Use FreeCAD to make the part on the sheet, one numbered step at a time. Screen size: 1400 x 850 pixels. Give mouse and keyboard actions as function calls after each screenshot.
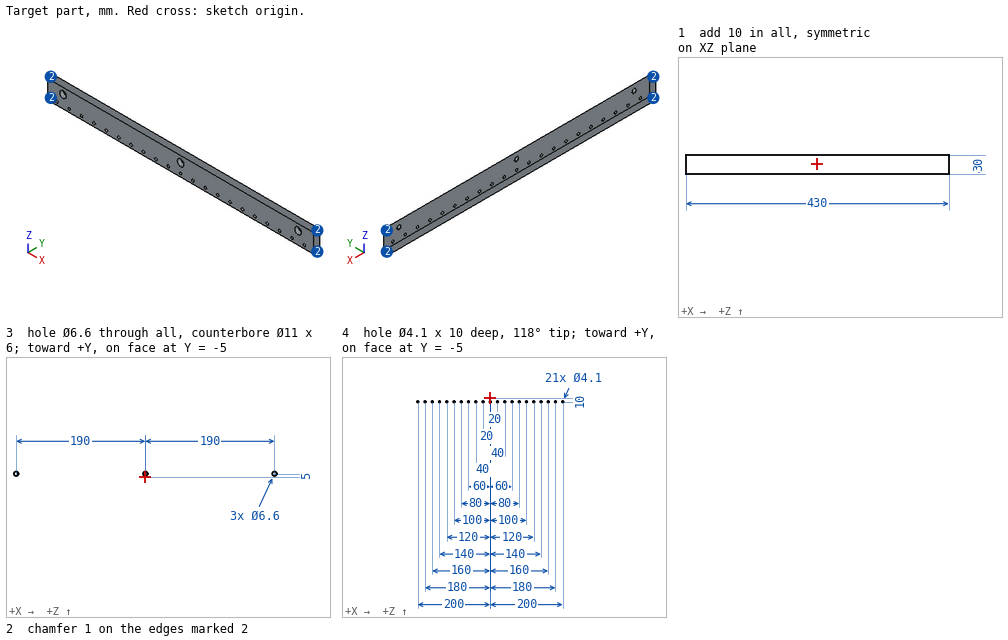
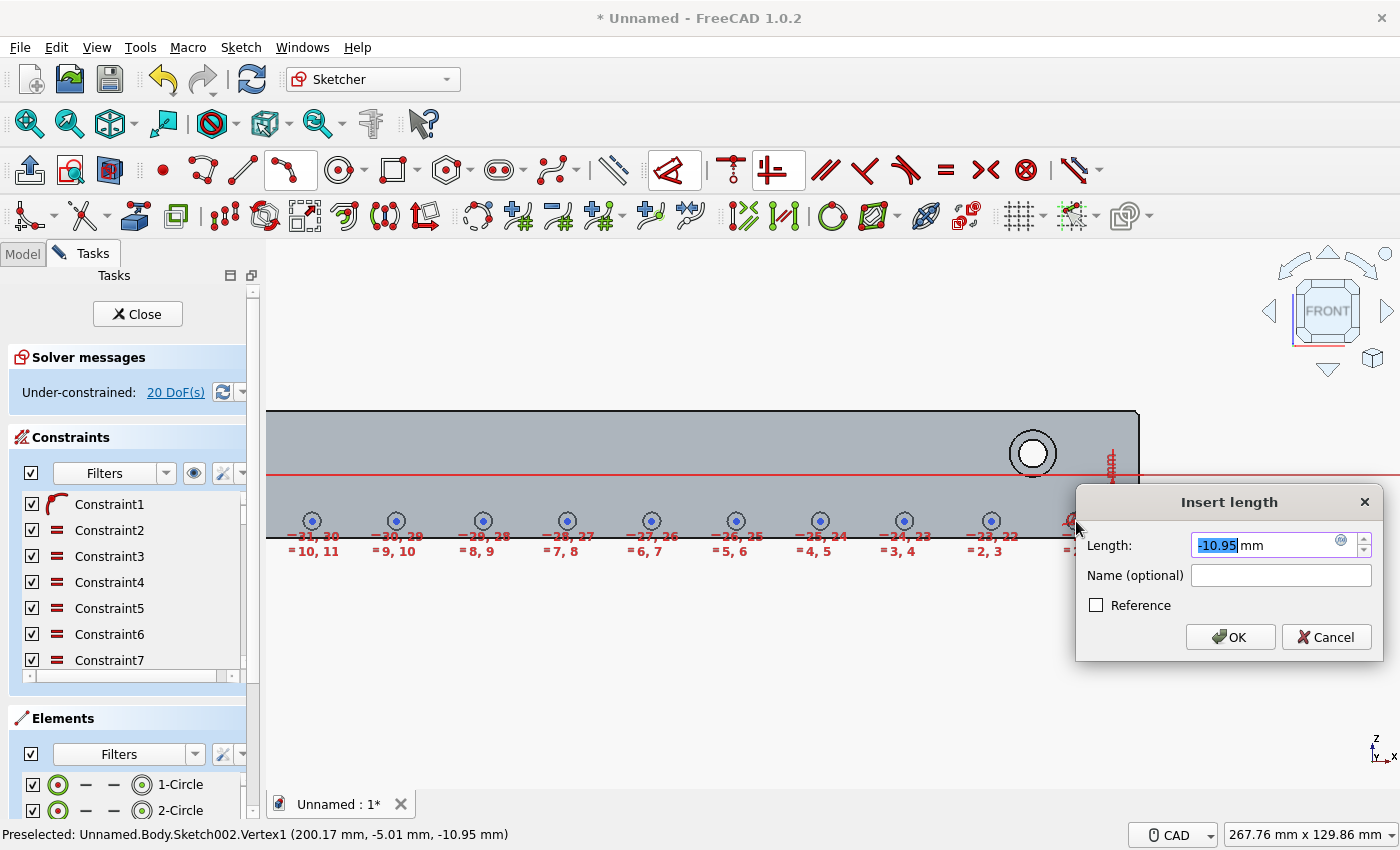
text(-10)
key(Return)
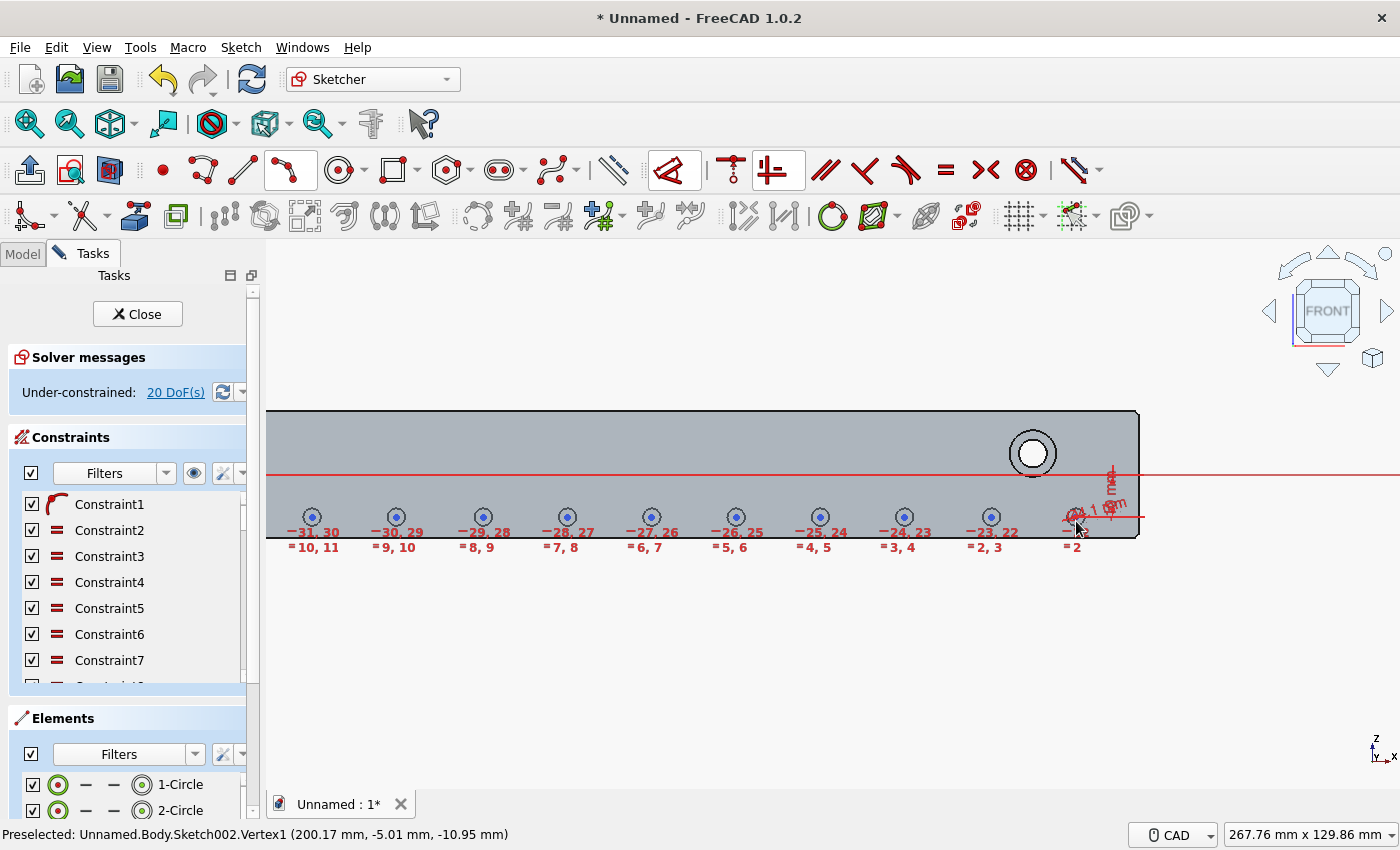
click(568, 517)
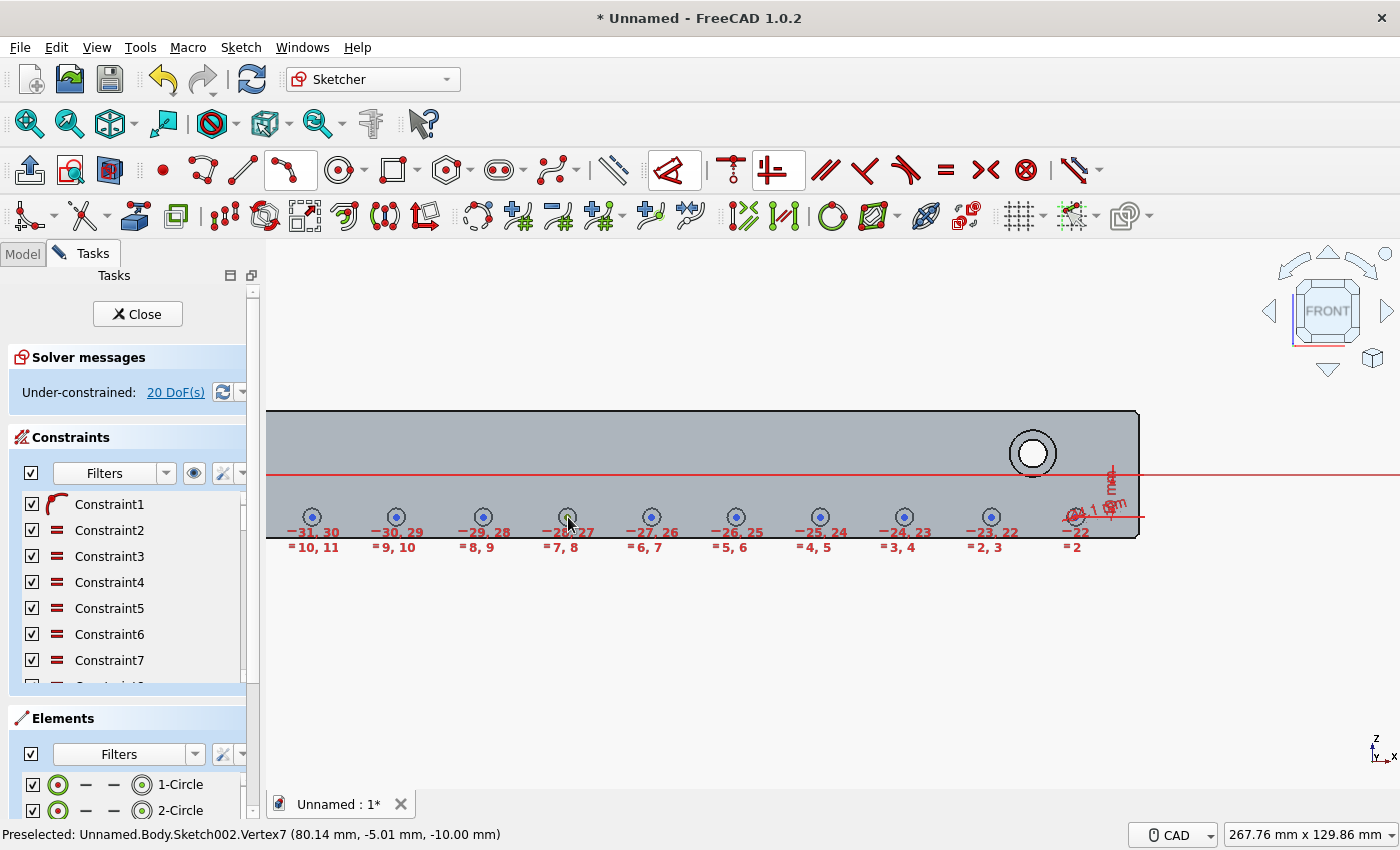
key(l)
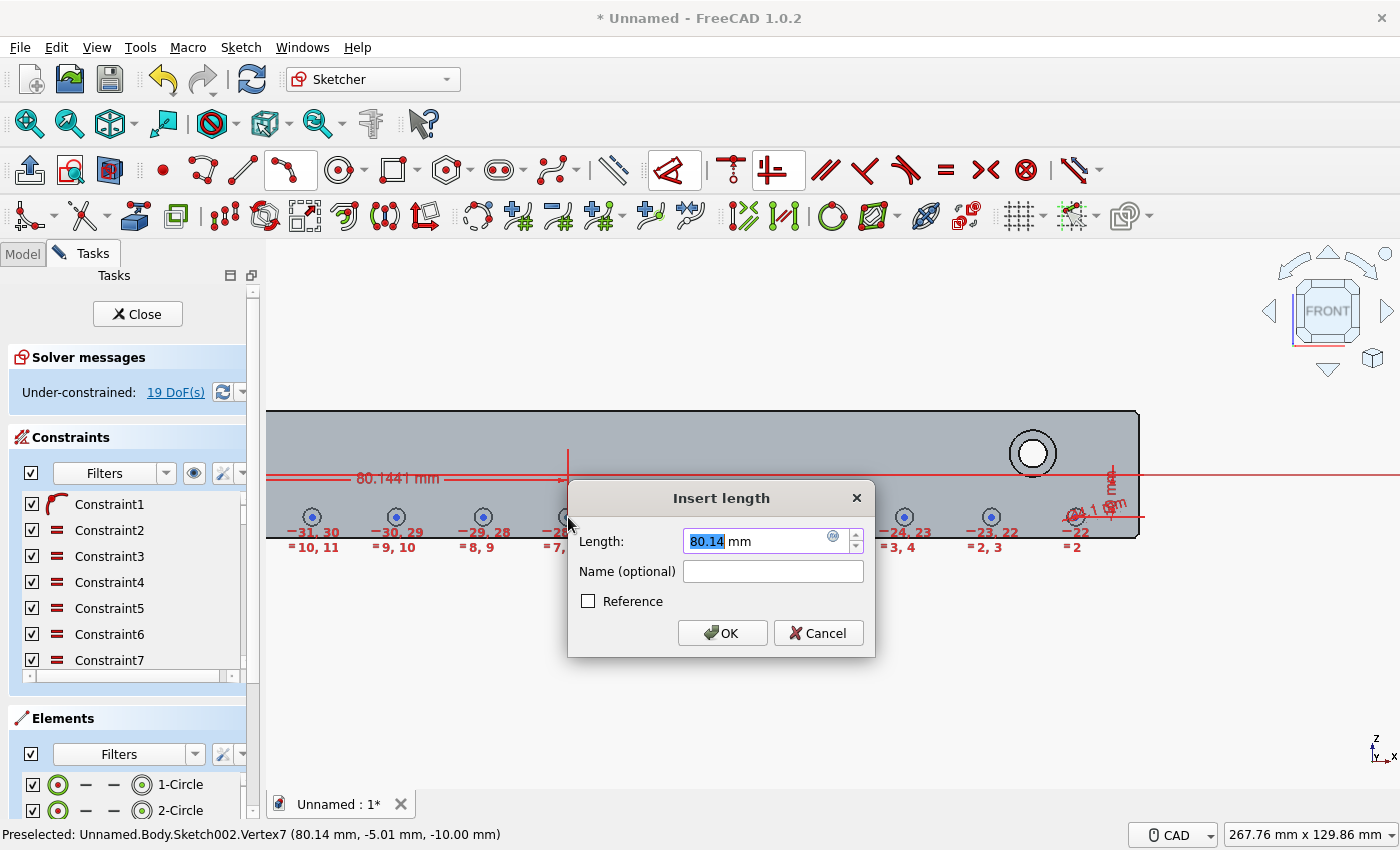
text(80)
key(Return)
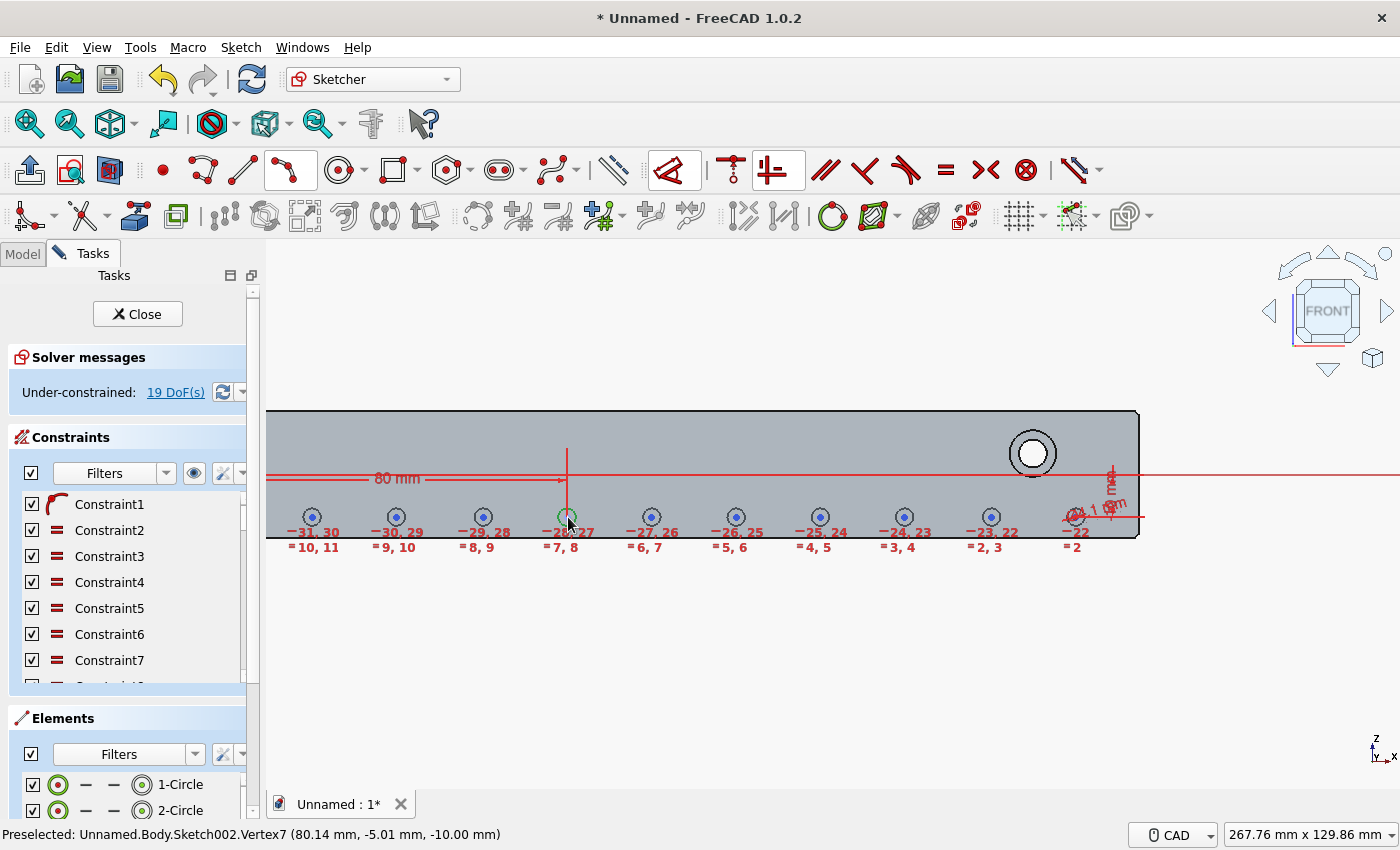
click(483, 517)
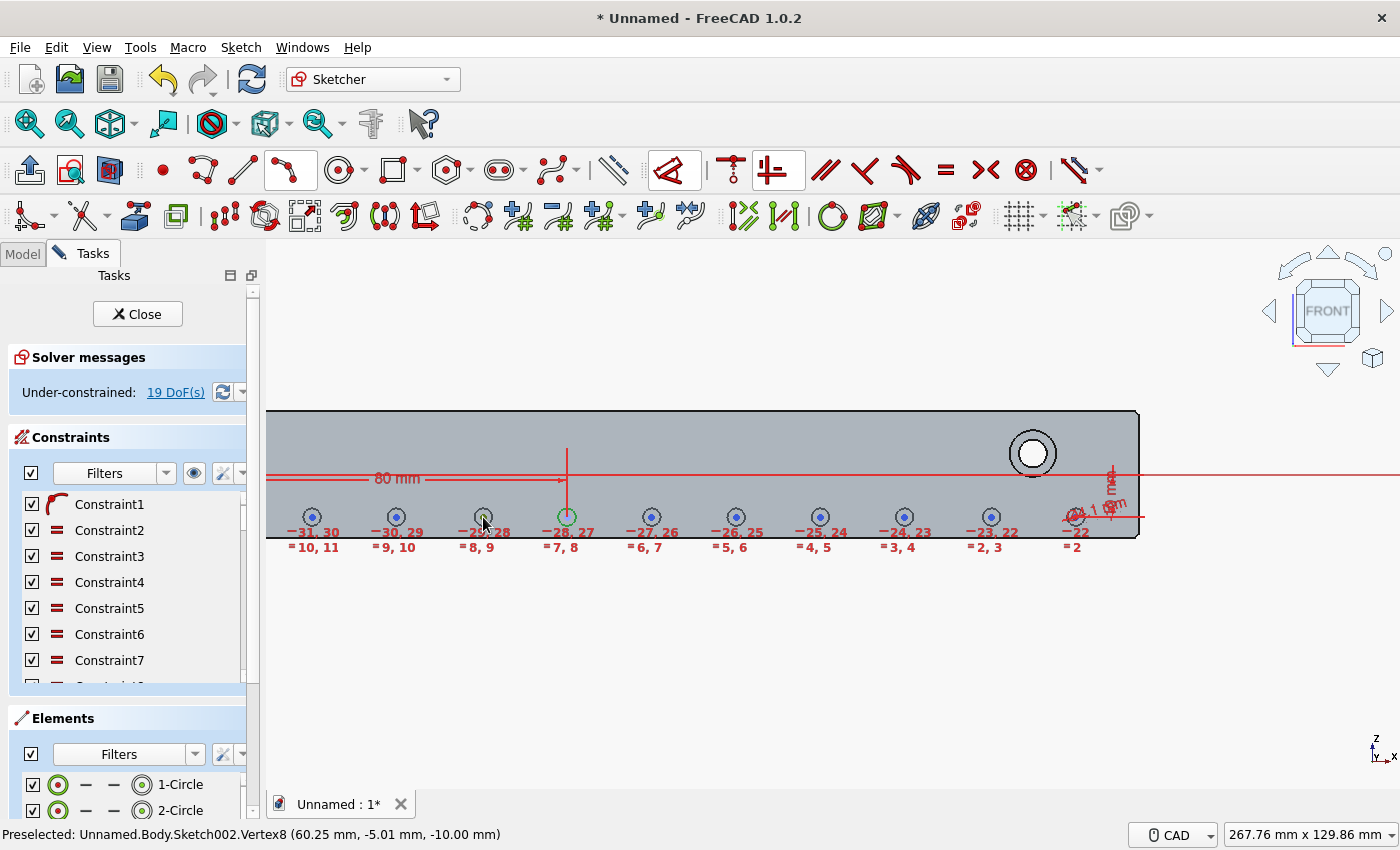
key(l)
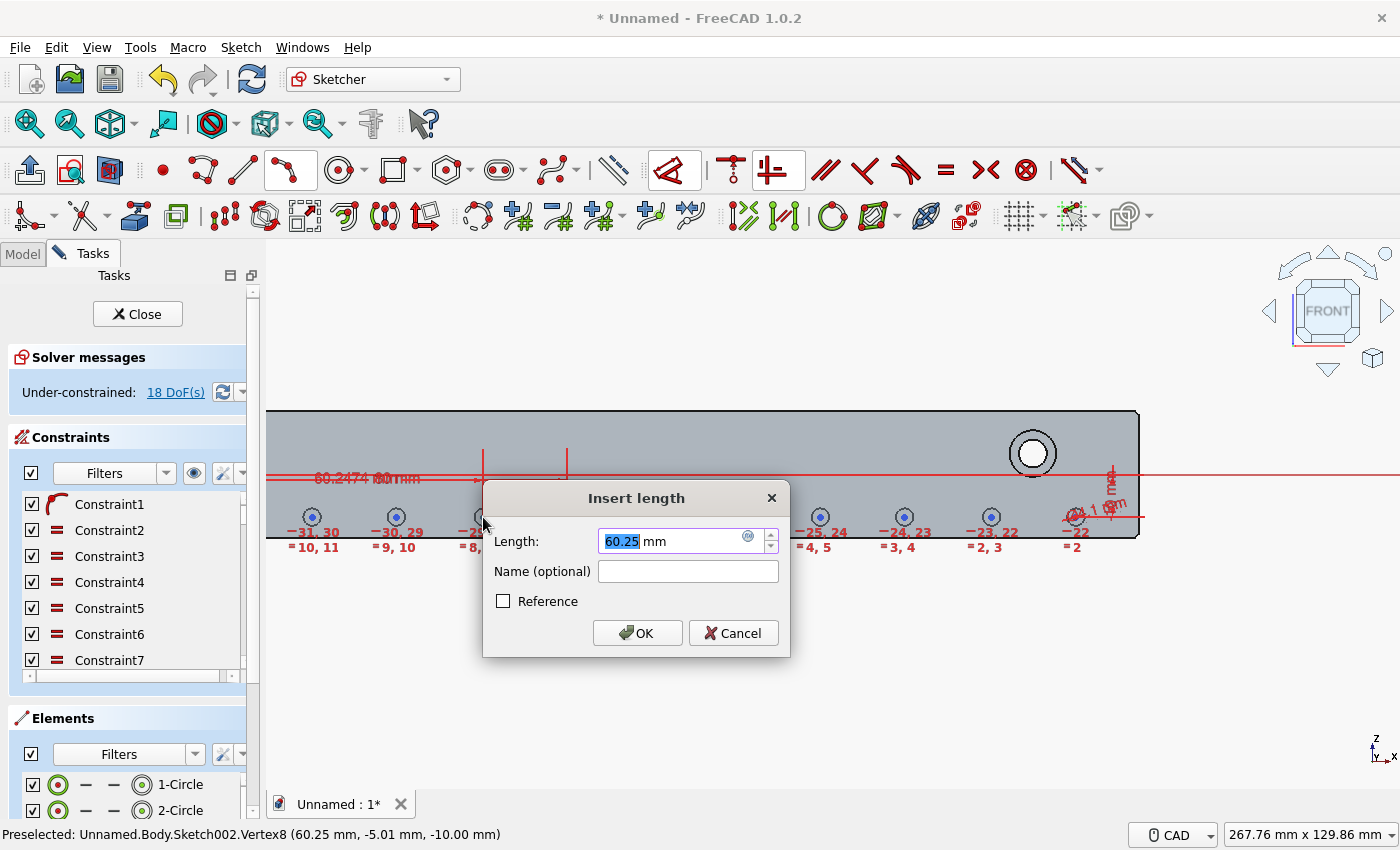
text(60)
key(Return)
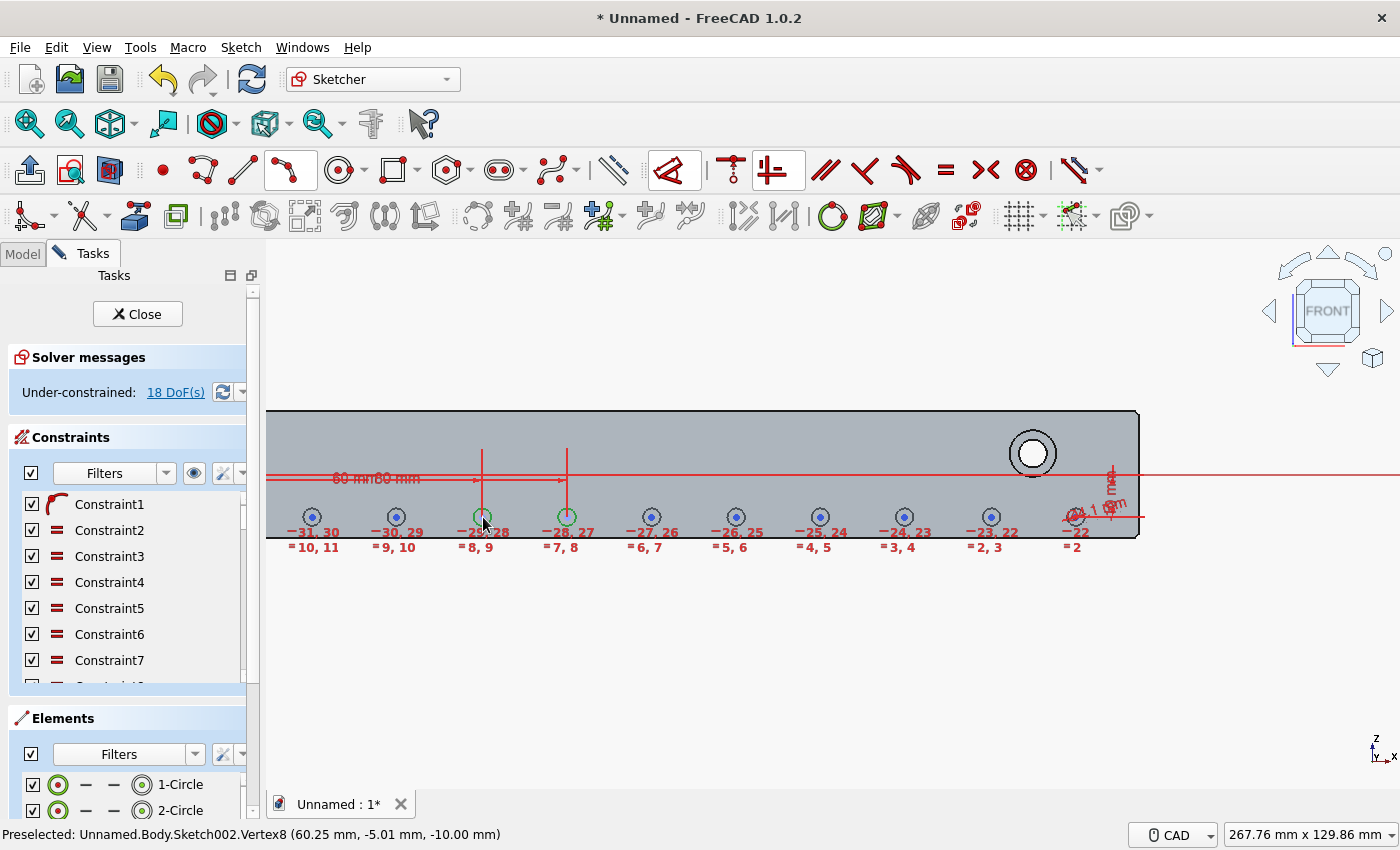
click(396, 517)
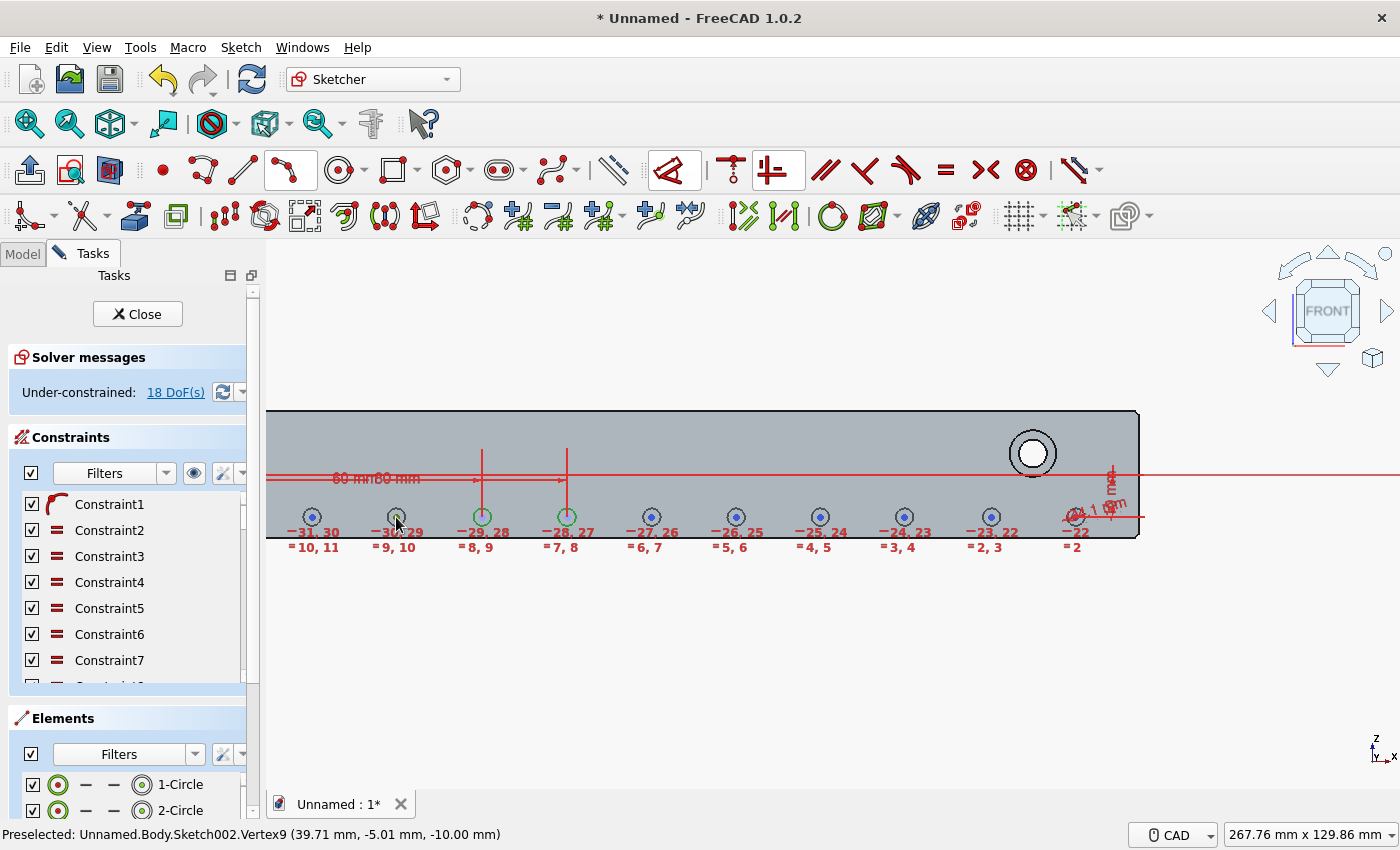
key(l)